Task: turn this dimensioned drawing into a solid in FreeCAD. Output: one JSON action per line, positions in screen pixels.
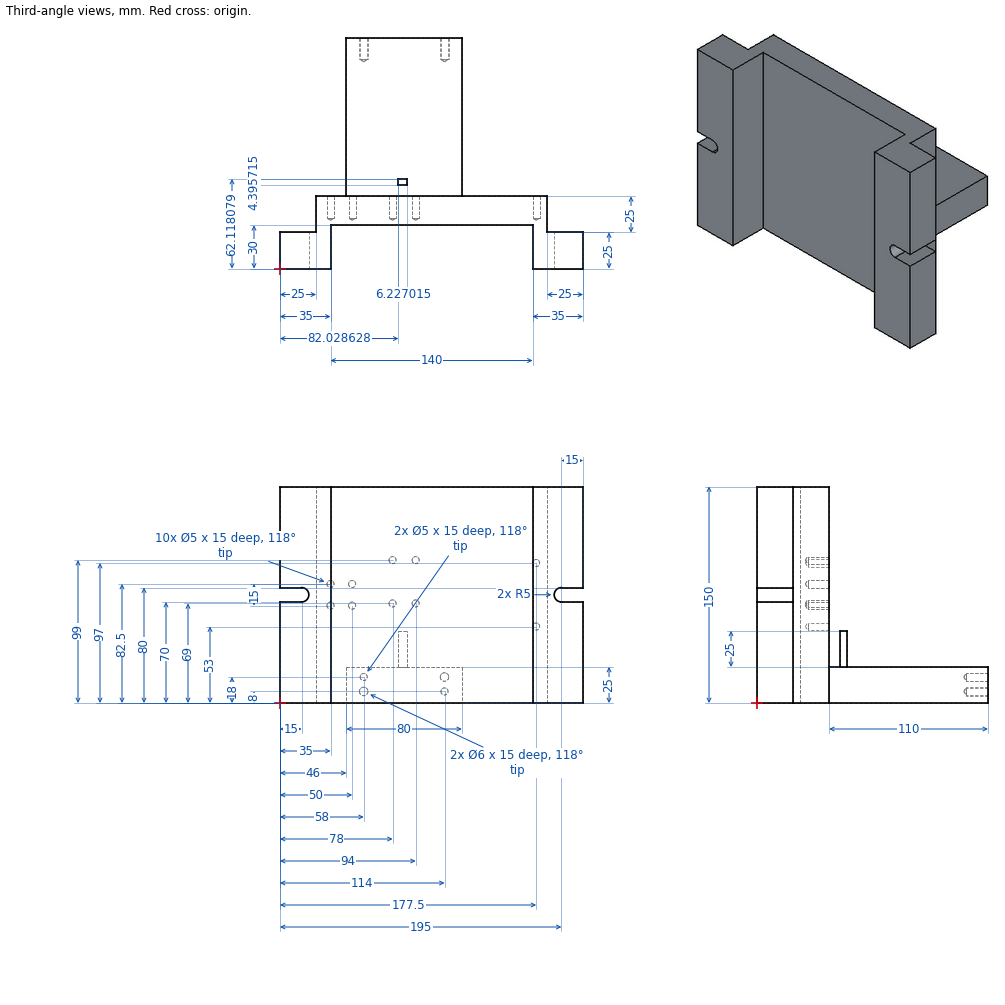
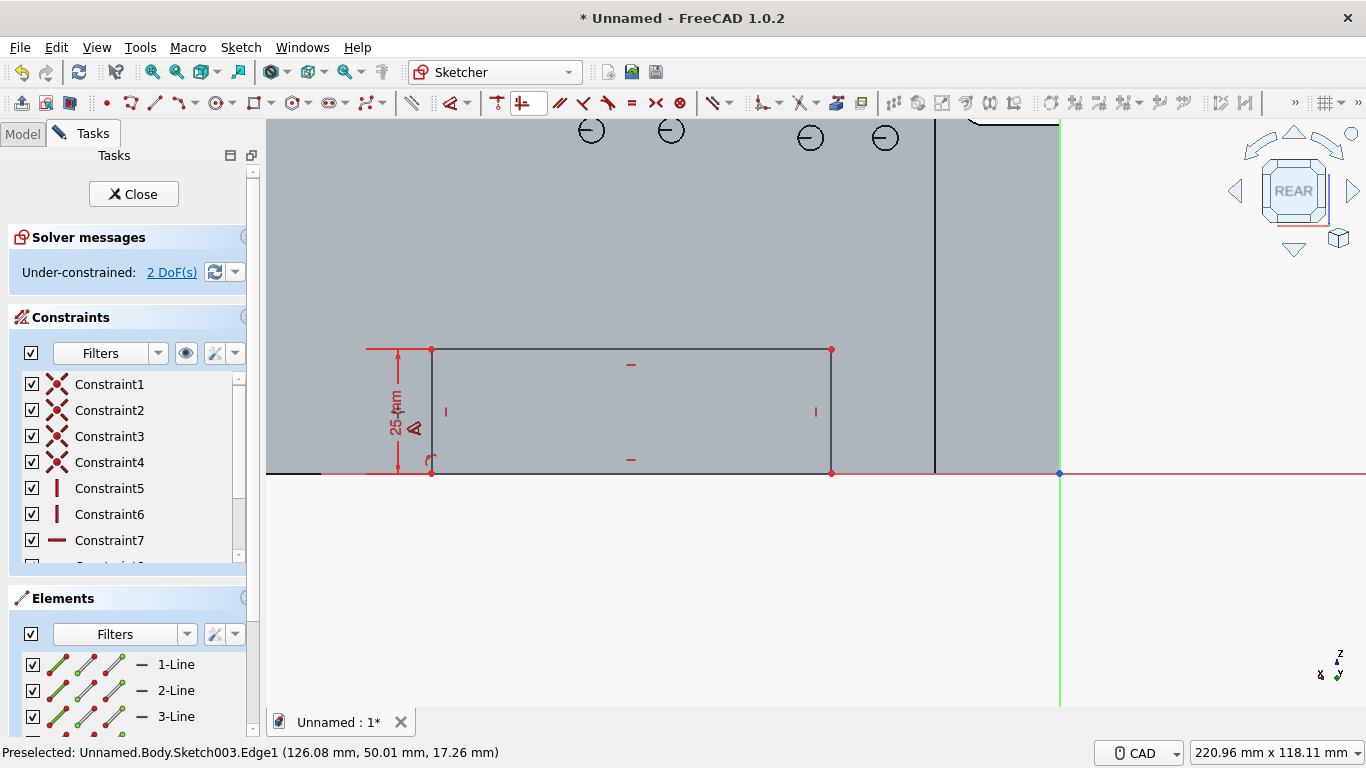
{"action": "left_click", "coordinate": [552, 474]}
{"action": "left_click", "coordinate": [632, 508]}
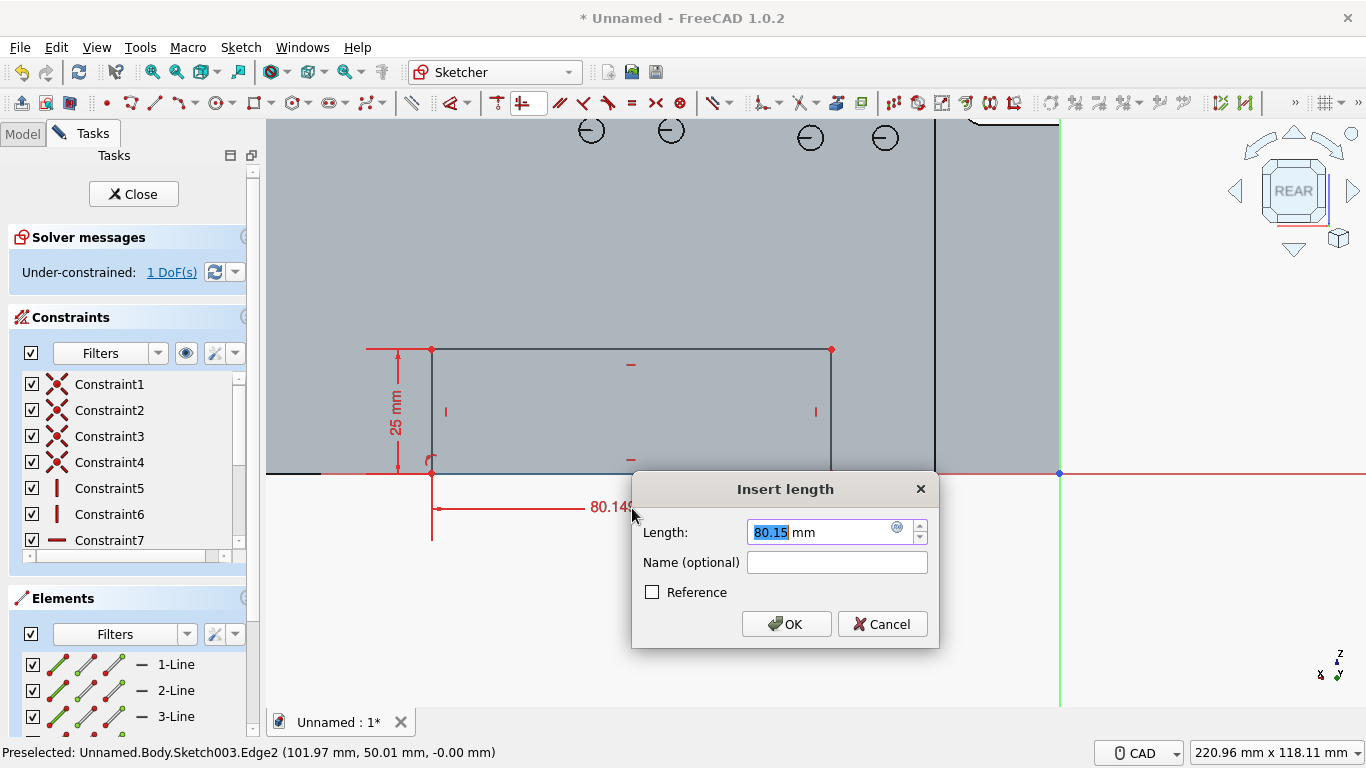
{"action": "type", "text": "80"}
{"action": "key", "text": "Return"}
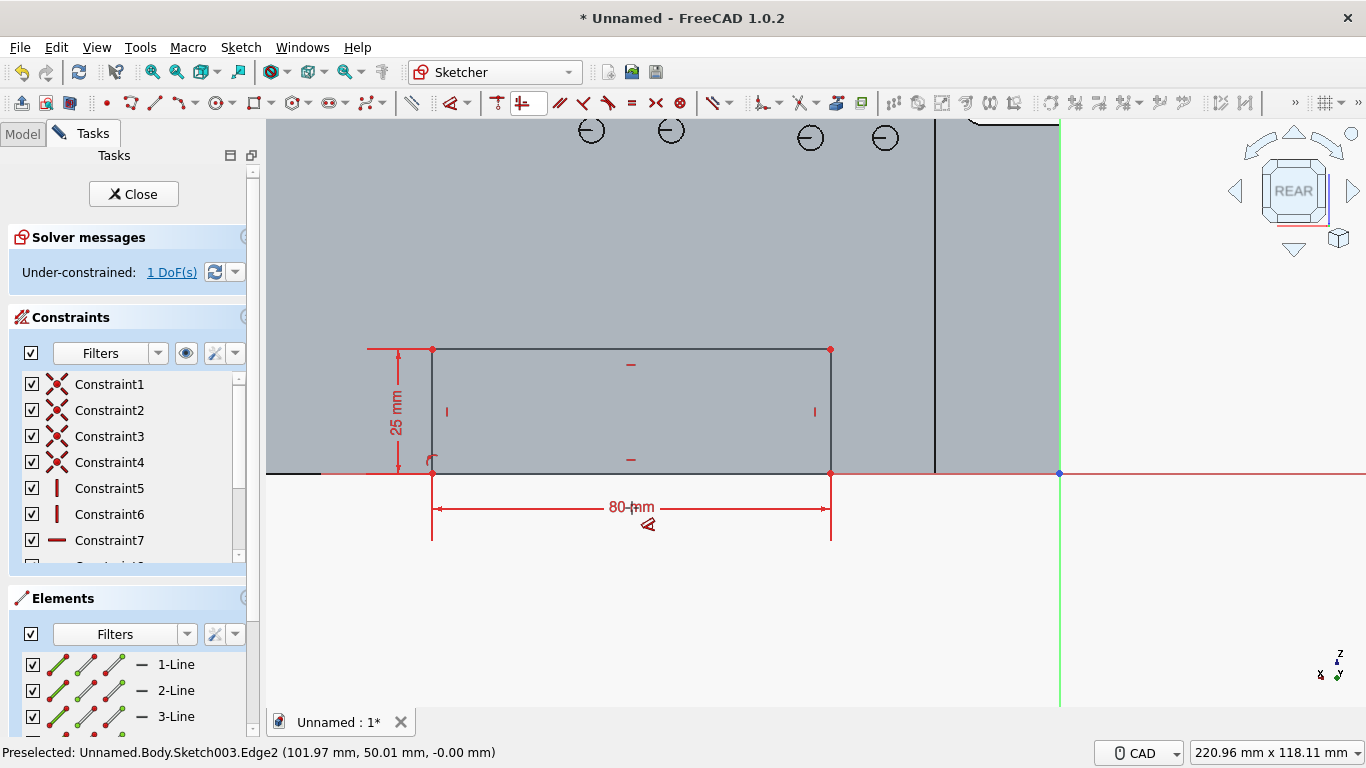
{"action": "left_click", "coordinate": [831, 474]}
{"action": "left_click", "coordinate": [945, 508]}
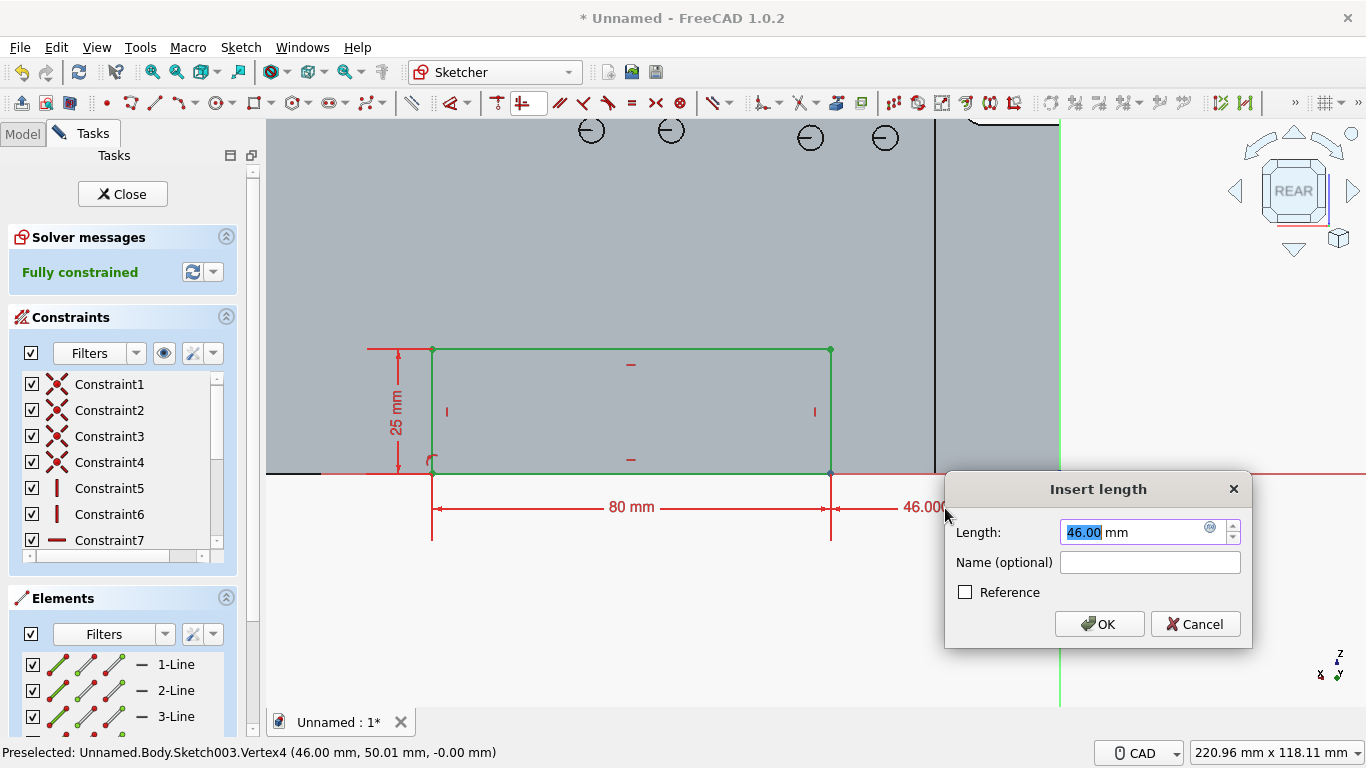
{"action": "type", "text": "46"}
{"action": "key", "text": "Return"}
{"action": "key", "text": "Escape"}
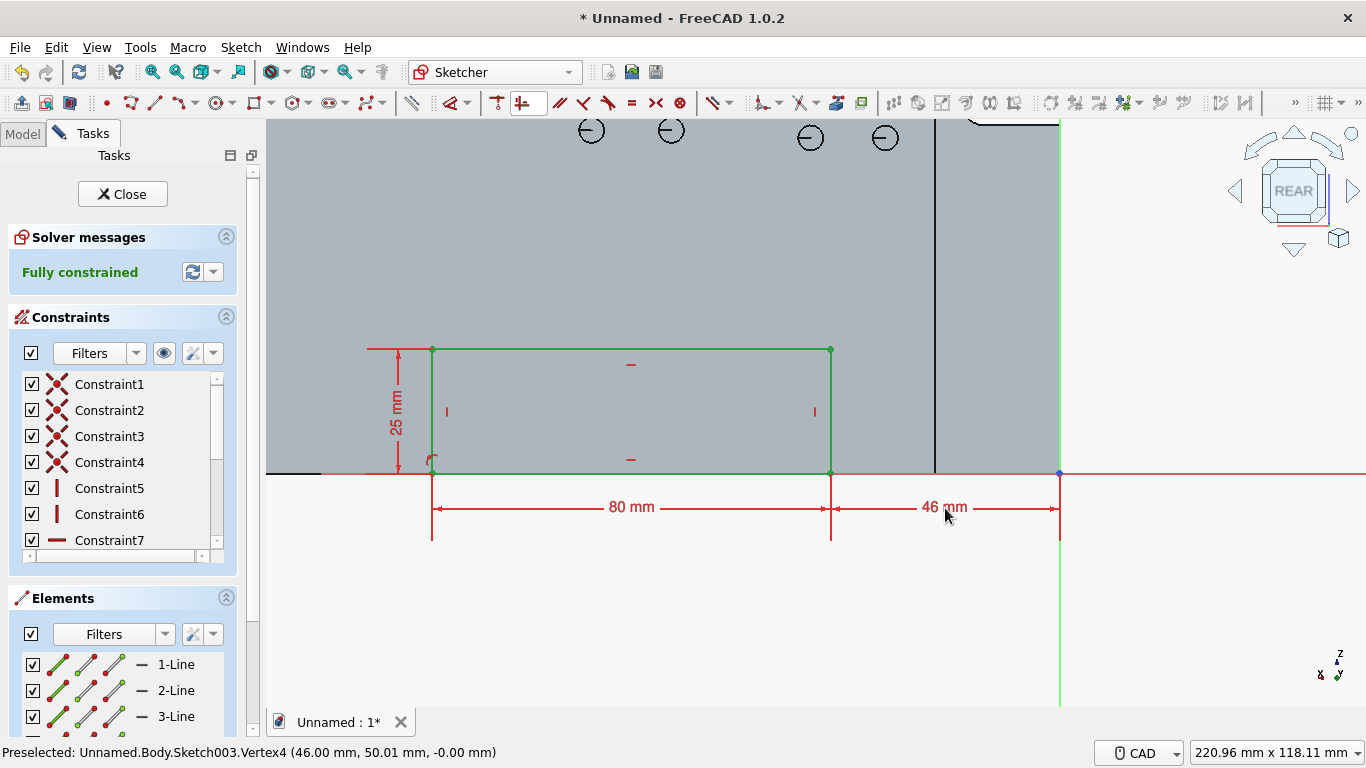
{"action": "left_click", "coordinate": [123, 194]}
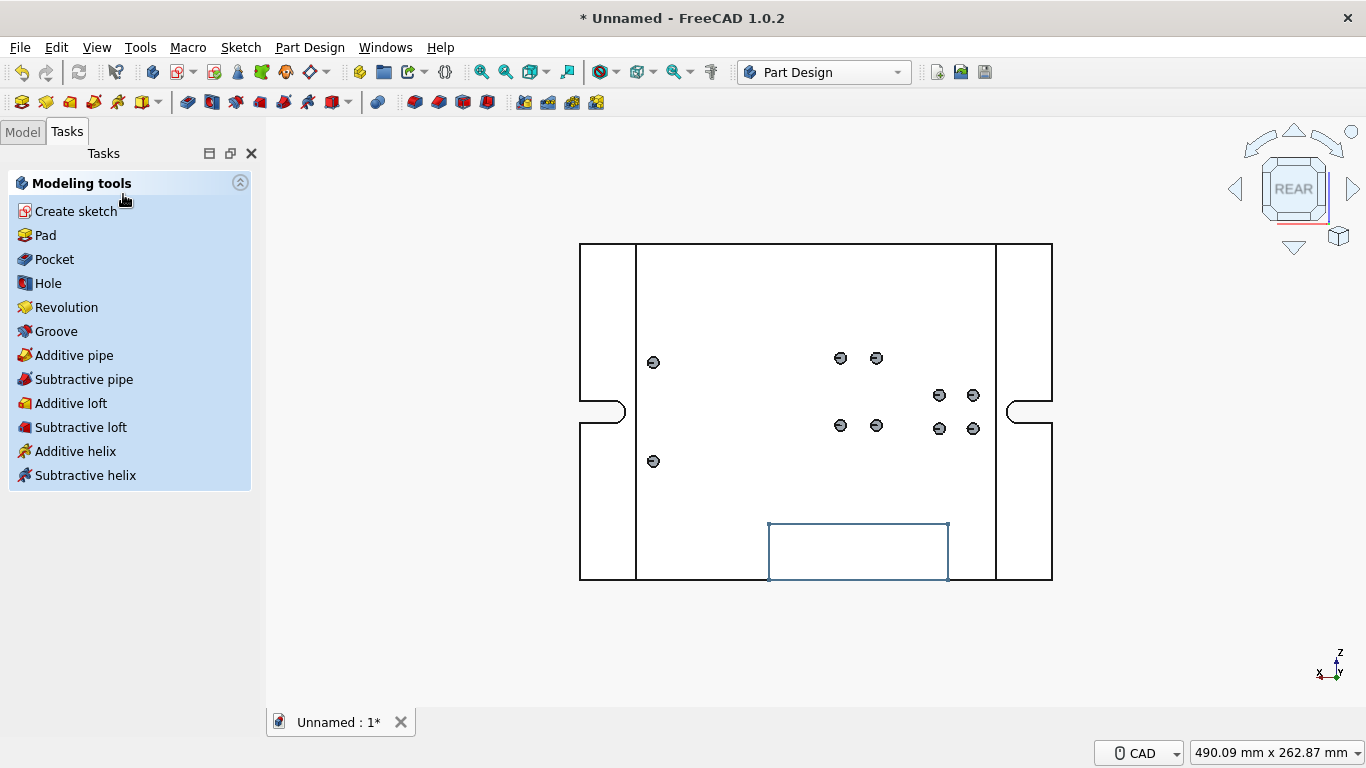
{"action": "left_click", "coordinate": [22, 102]}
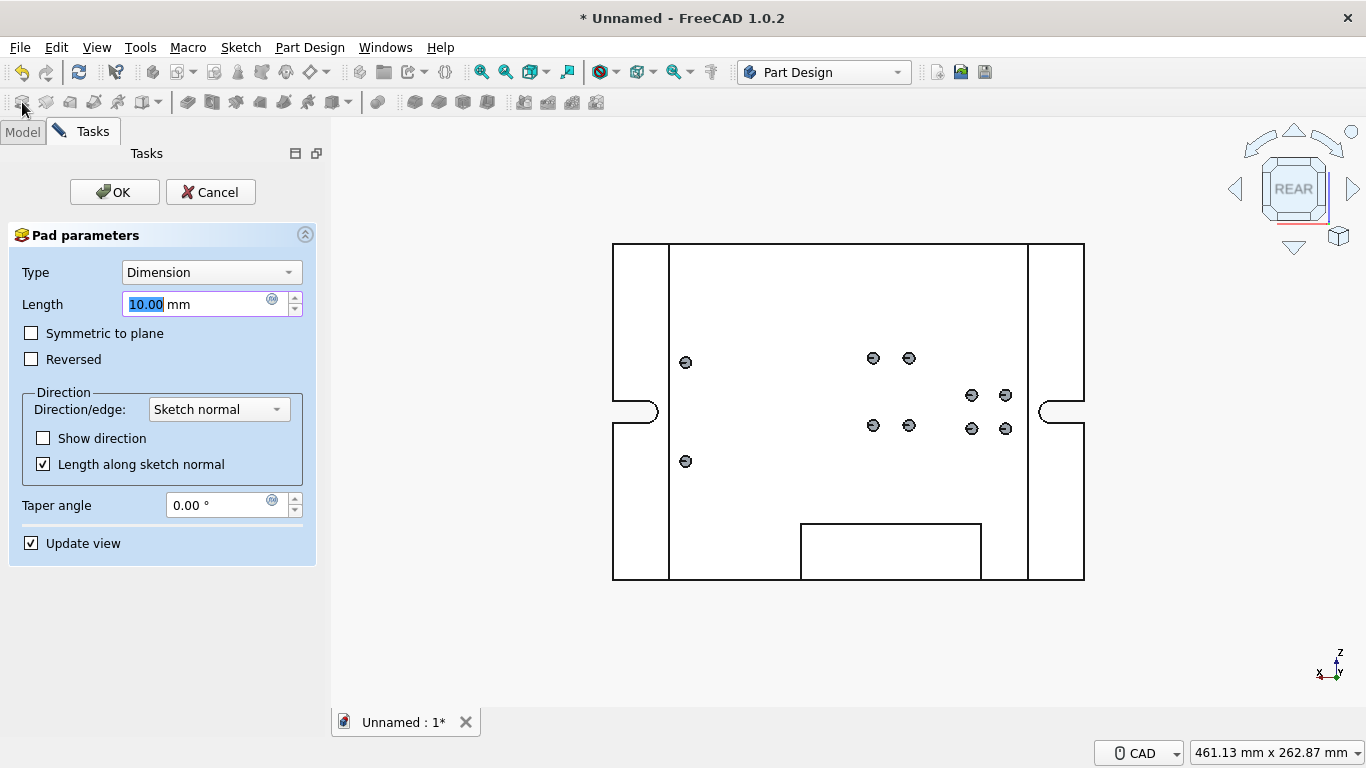
{"action": "type", "text": "110"}
{"action": "key", "text": "Tab"}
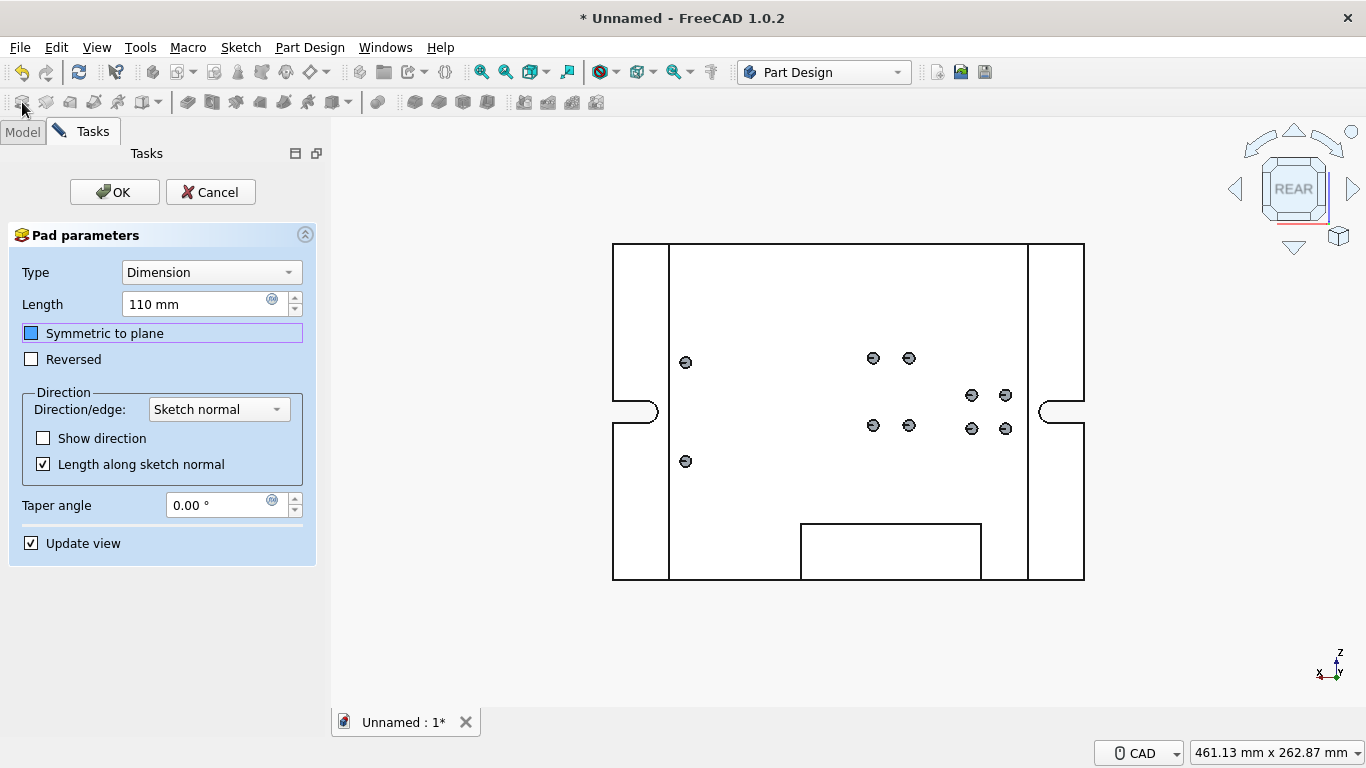
{"action": "left_click", "coordinate": [115, 192]}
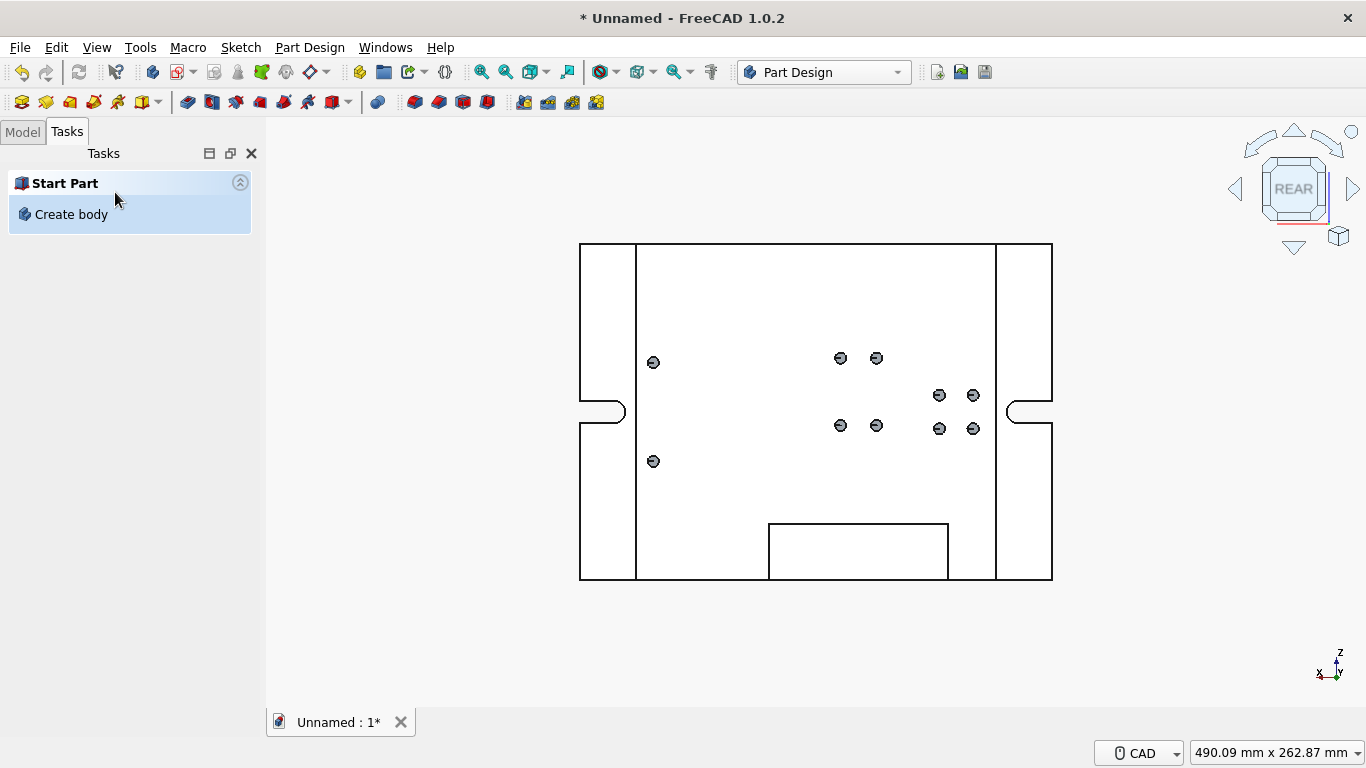
{"action": "left_click", "coordinate": [807, 551]}